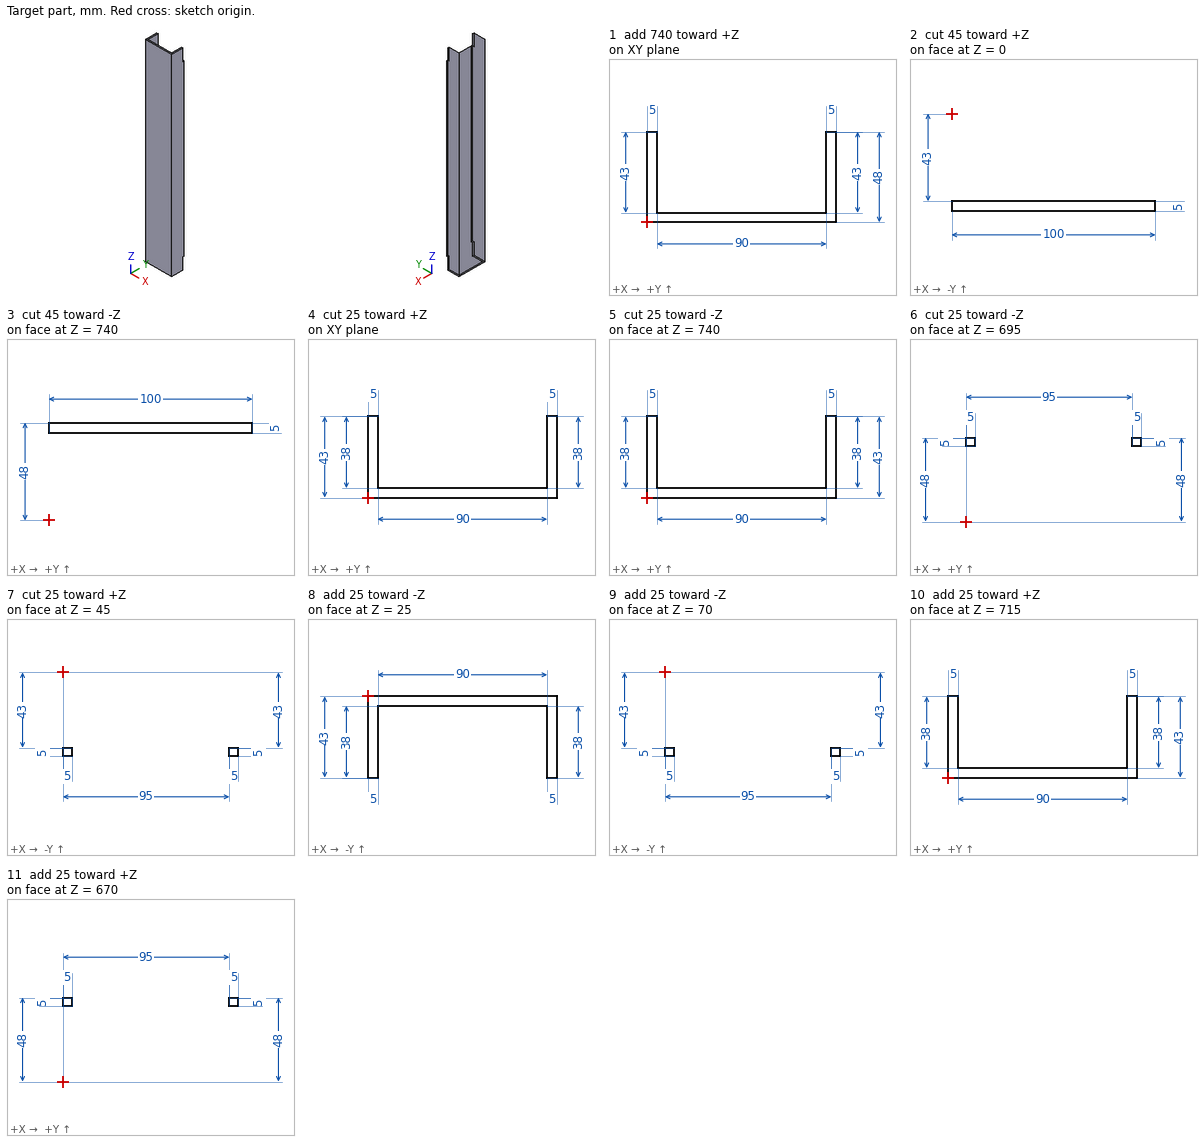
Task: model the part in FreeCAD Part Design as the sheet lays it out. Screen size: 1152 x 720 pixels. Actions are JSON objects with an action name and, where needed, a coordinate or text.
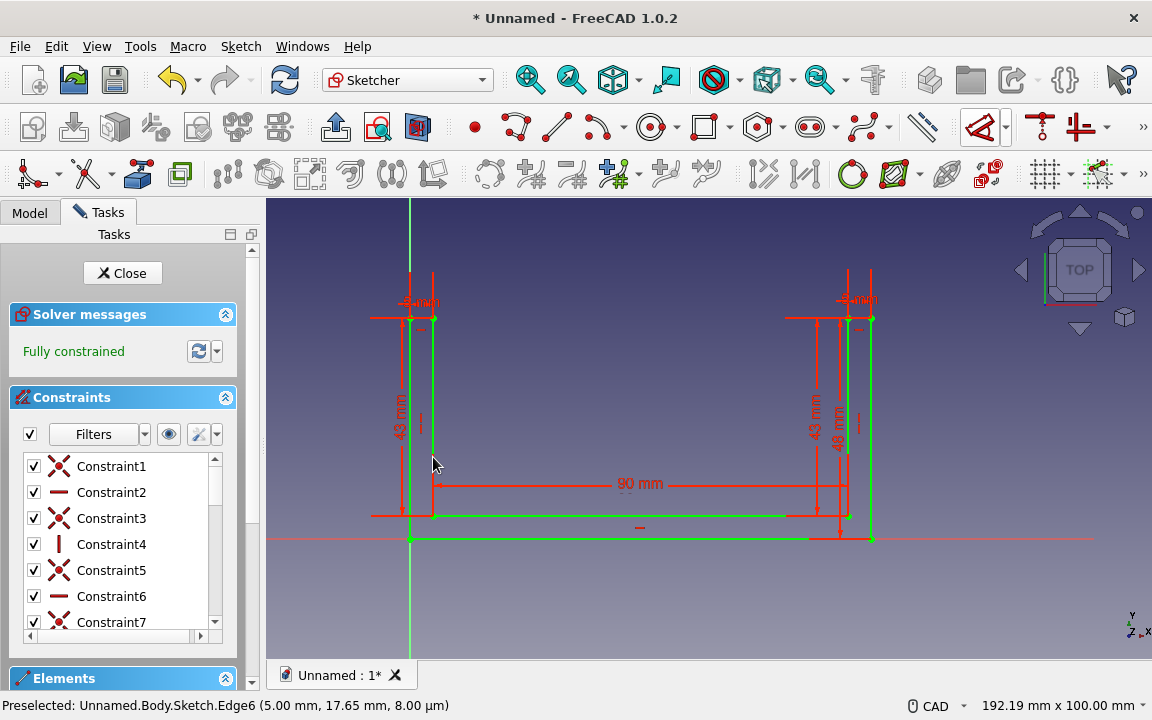
{"action": "left_click", "coordinate": [123, 273]}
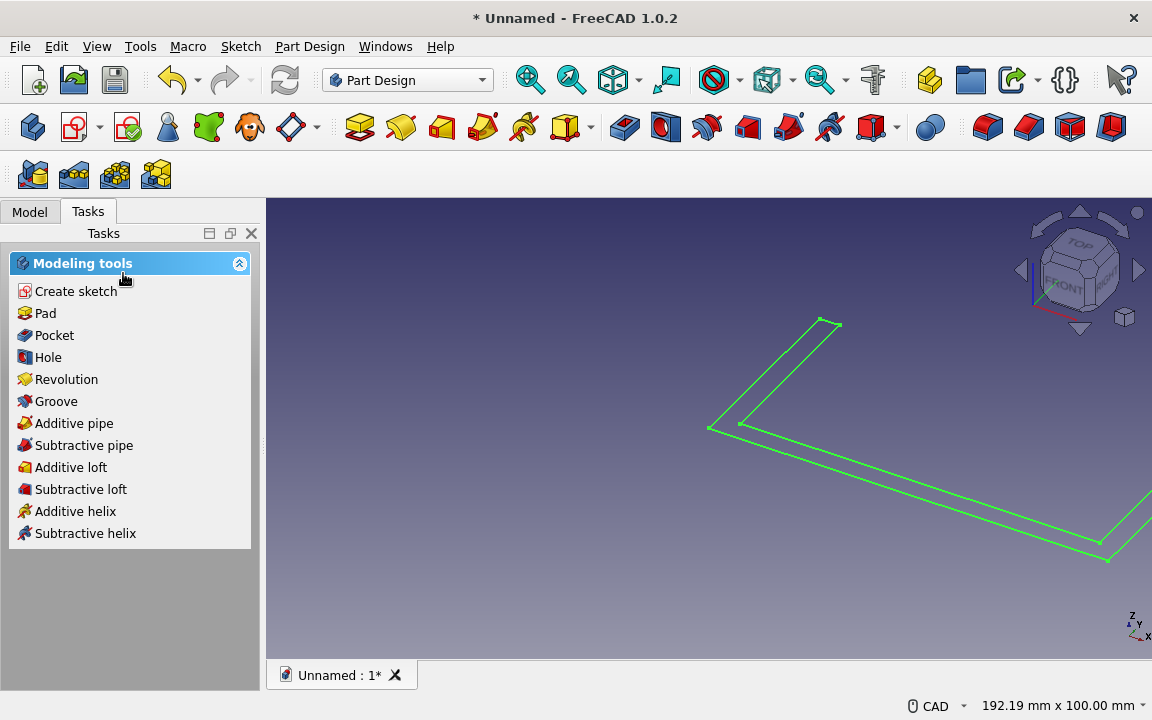
{"action": "left_click", "coordinate": [360, 128]}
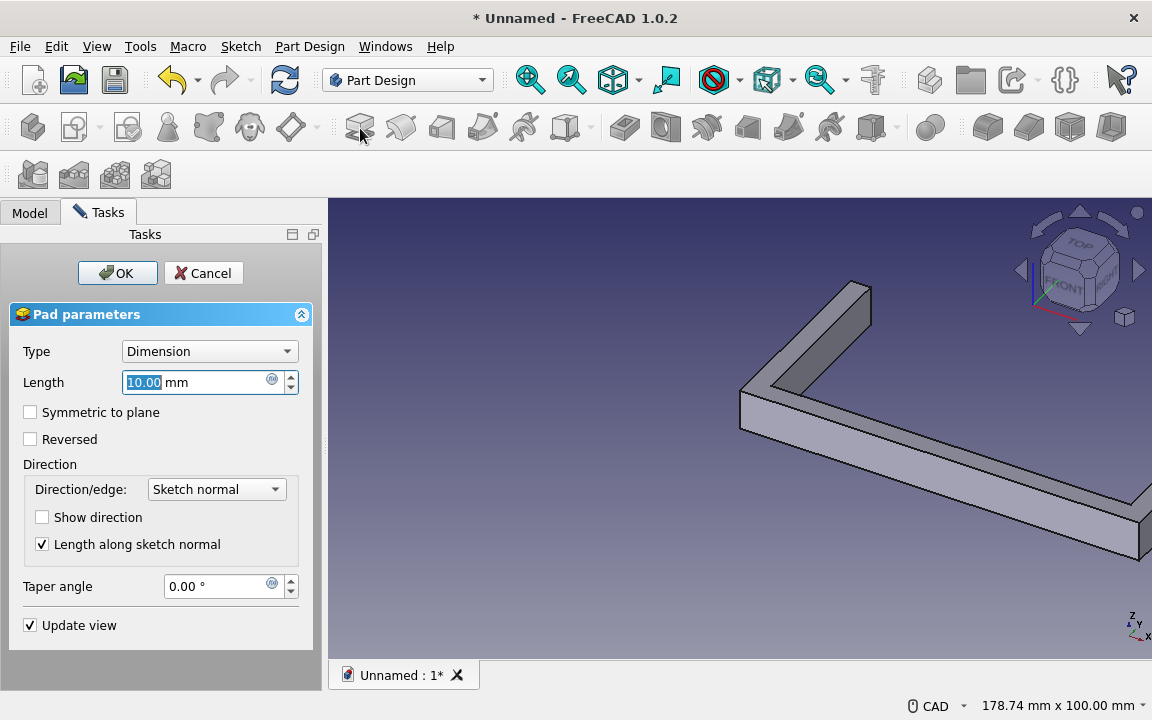
{"action": "type", "text": "740"}
{"action": "key", "text": "Tab"}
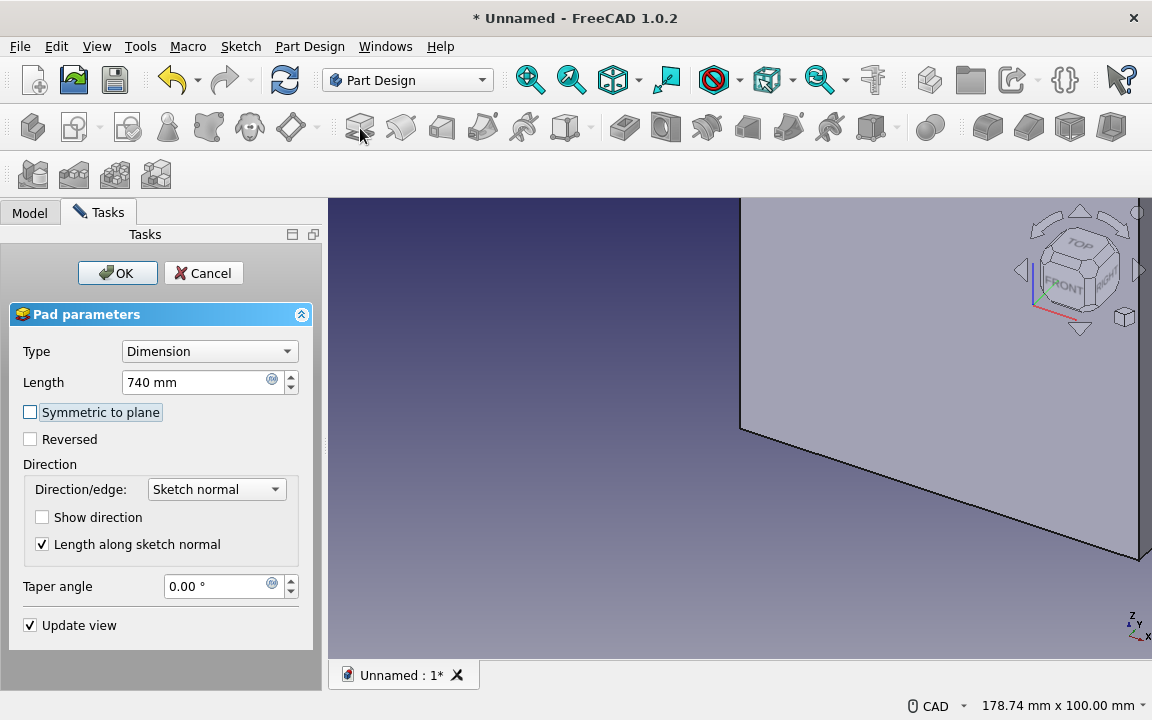
{"action": "left_click", "coordinate": [118, 273]}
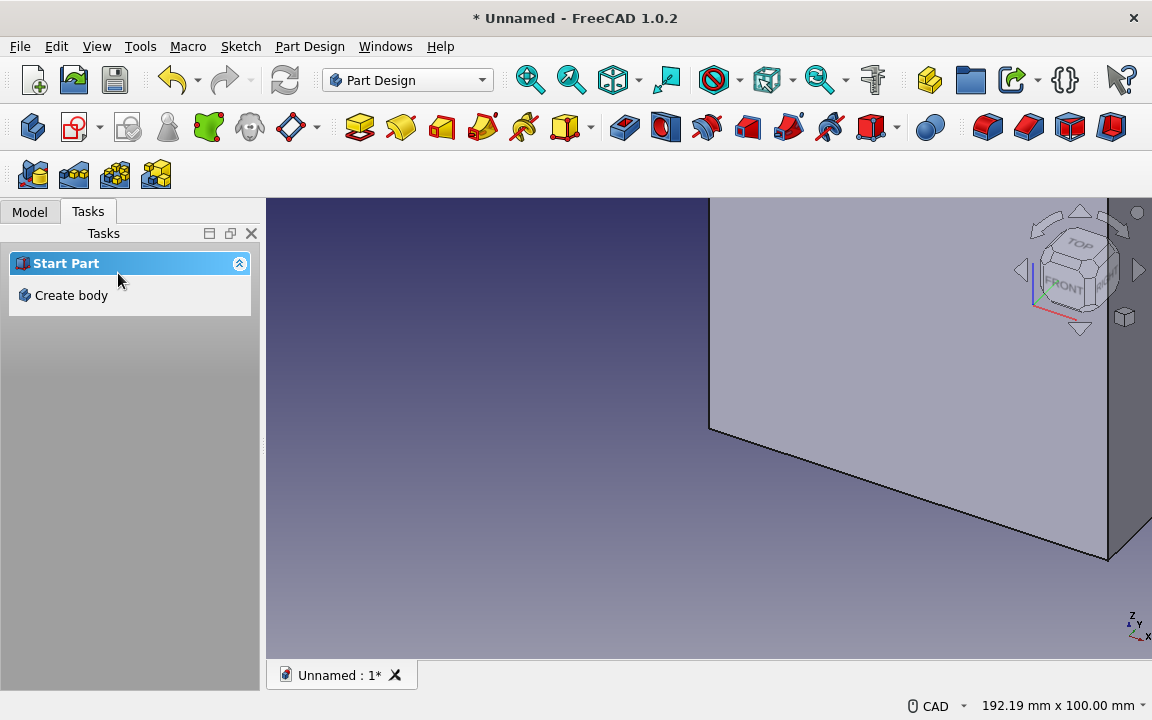
{"action": "left_click", "coordinate": [531, 80]}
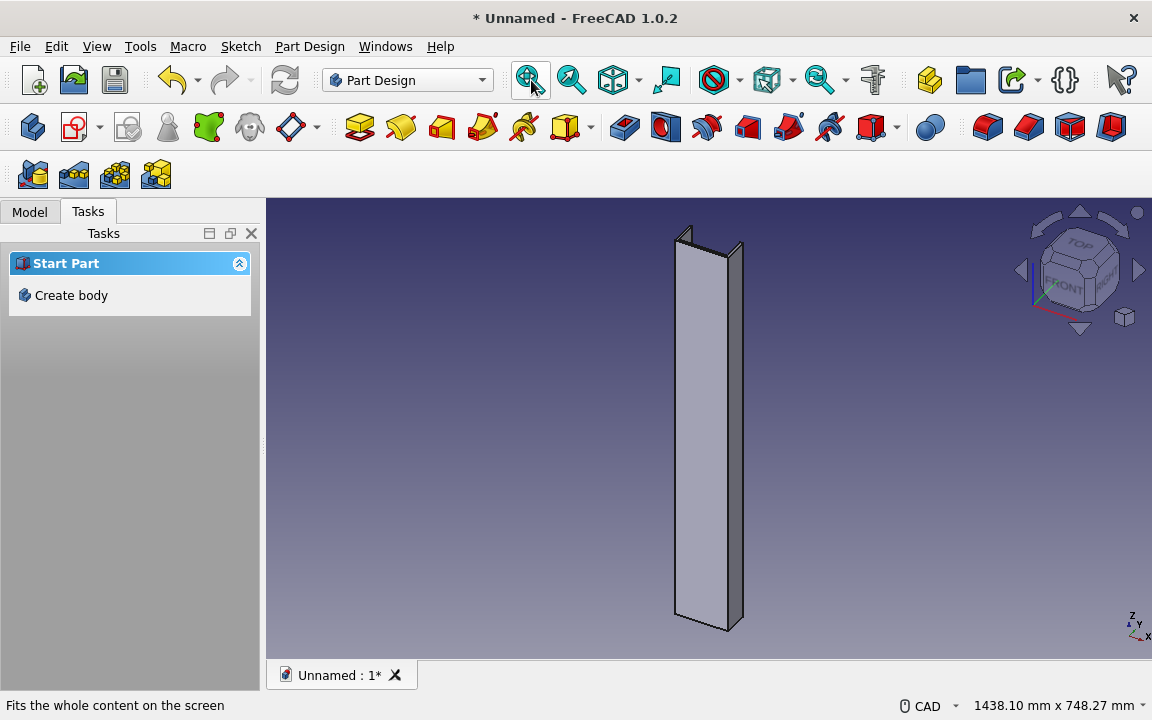
{"action": "key", "text": "5"}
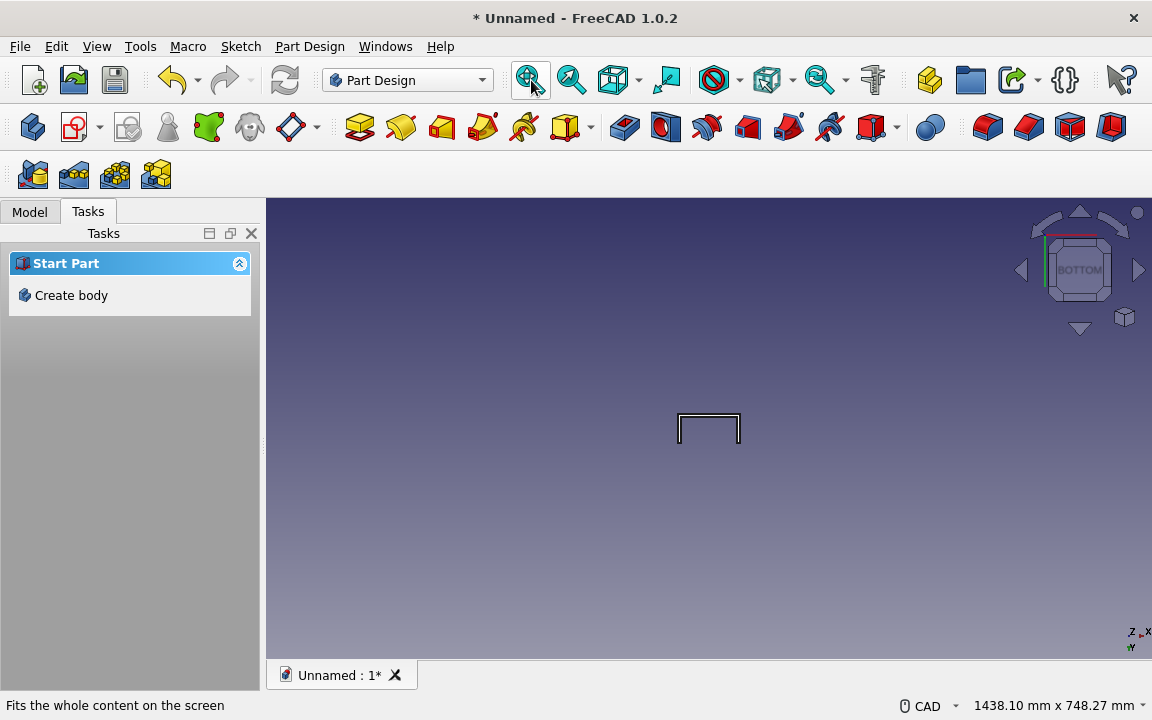
{"action": "left_click", "coordinate": [531, 80]}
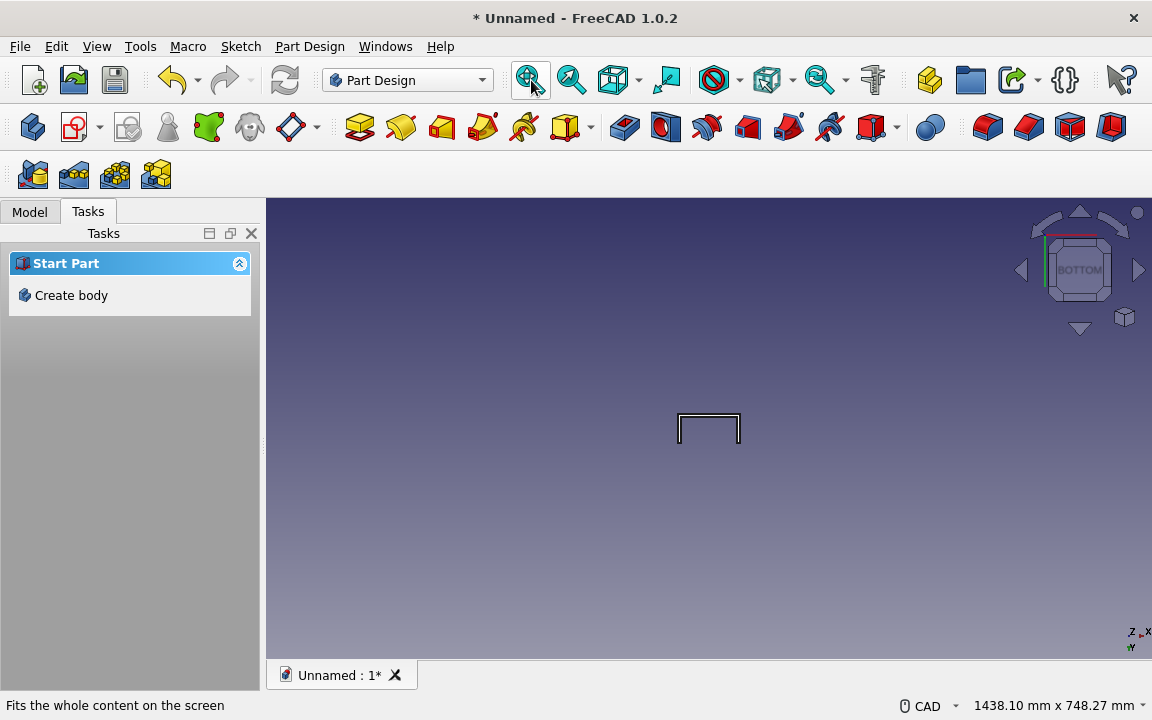
{"action": "scroll", "coordinate": [735, 415], "scroll_direction": "up", "scroll_amount": 13}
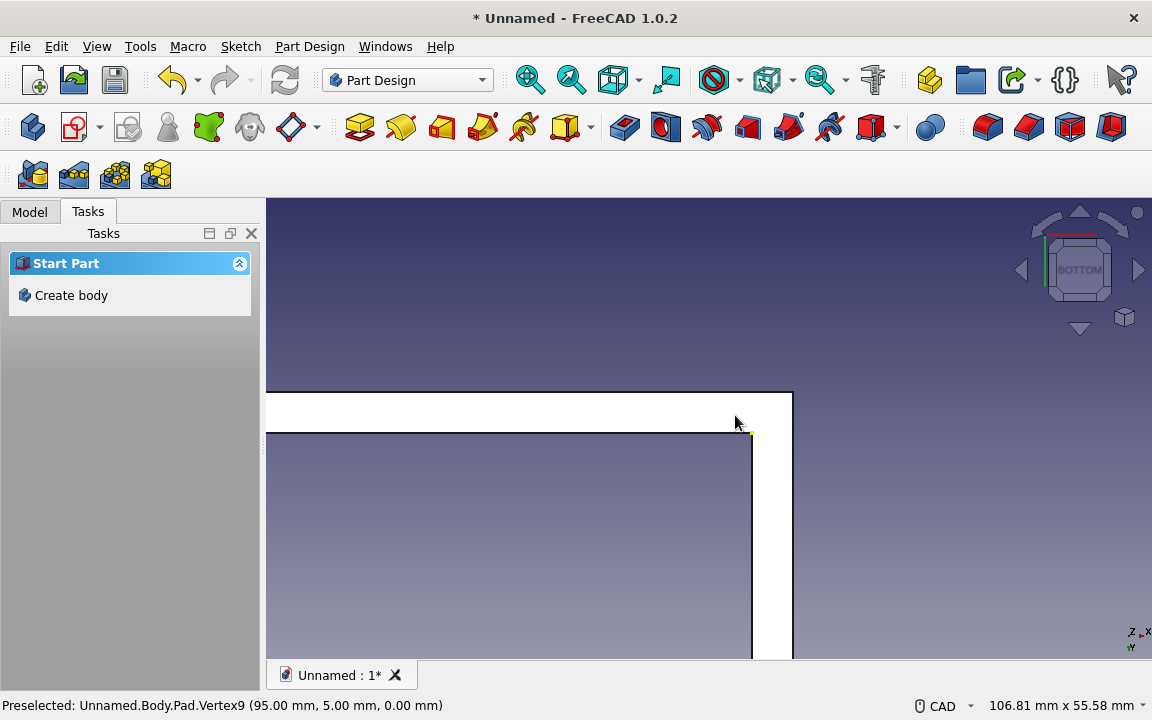
{"action": "left_click", "coordinate": [734, 419]}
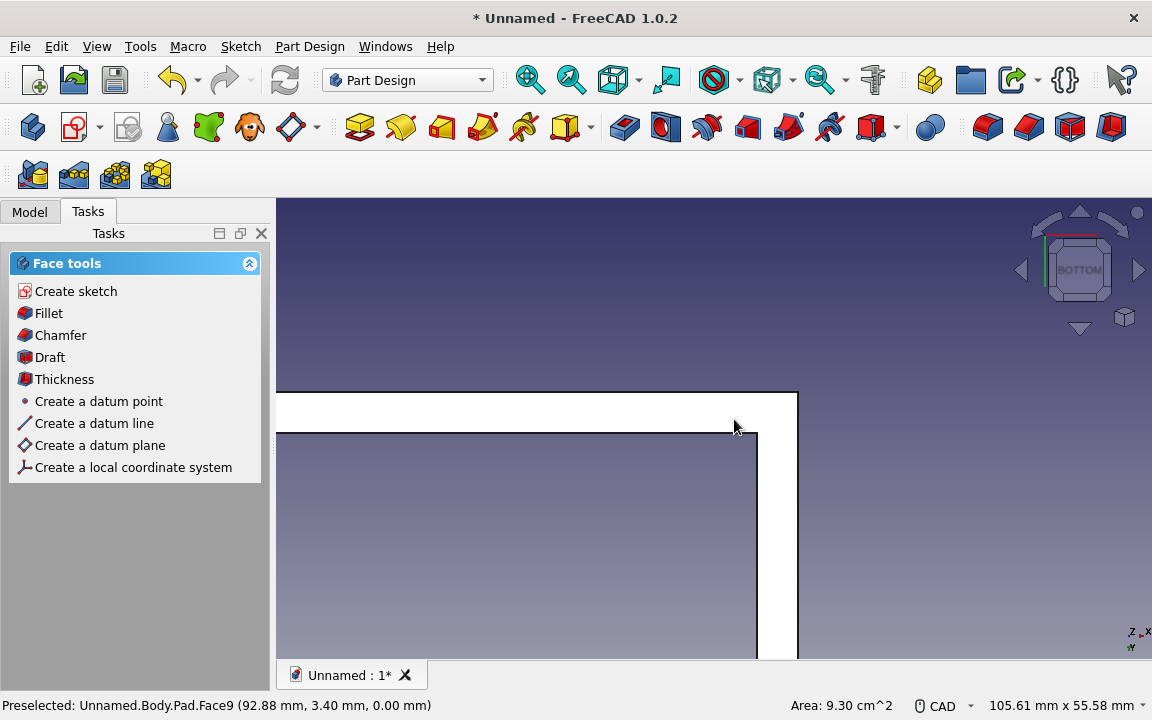
{"action": "left_click", "coordinate": [74, 128]}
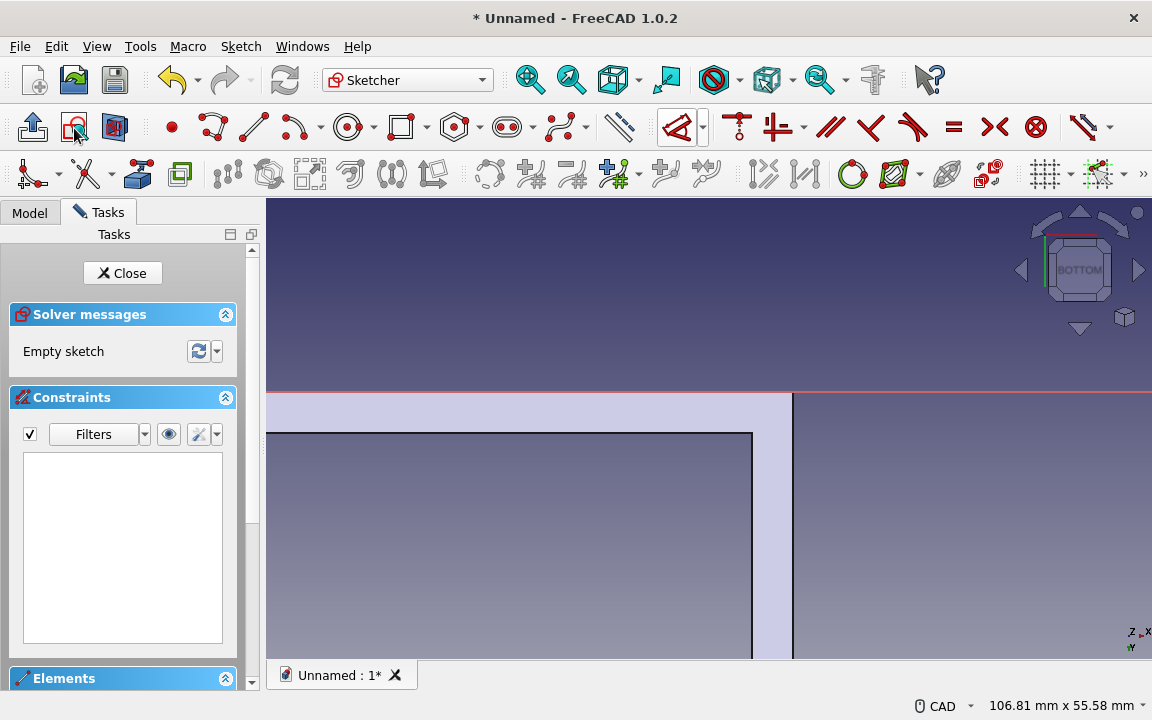
{"action": "scroll", "coordinate": [959, 231], "scroll_direction": "down", "scroll_amount": 3}